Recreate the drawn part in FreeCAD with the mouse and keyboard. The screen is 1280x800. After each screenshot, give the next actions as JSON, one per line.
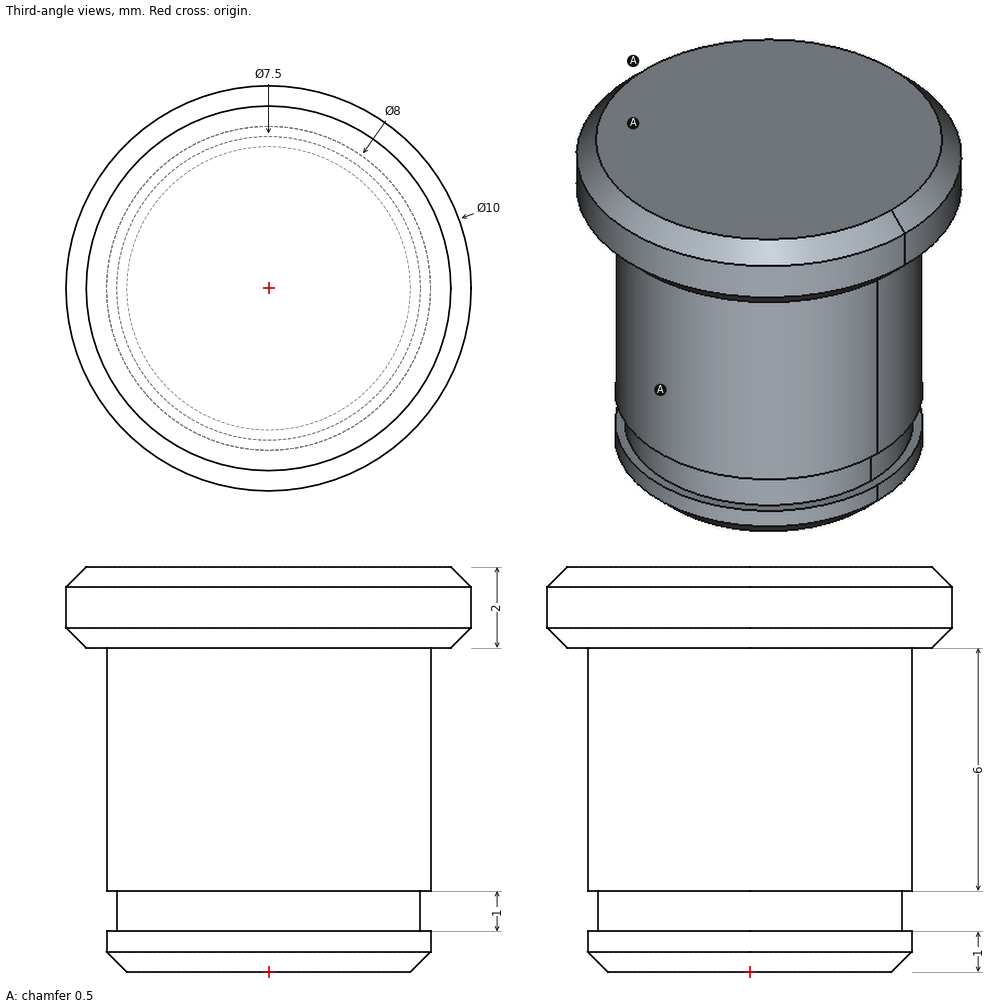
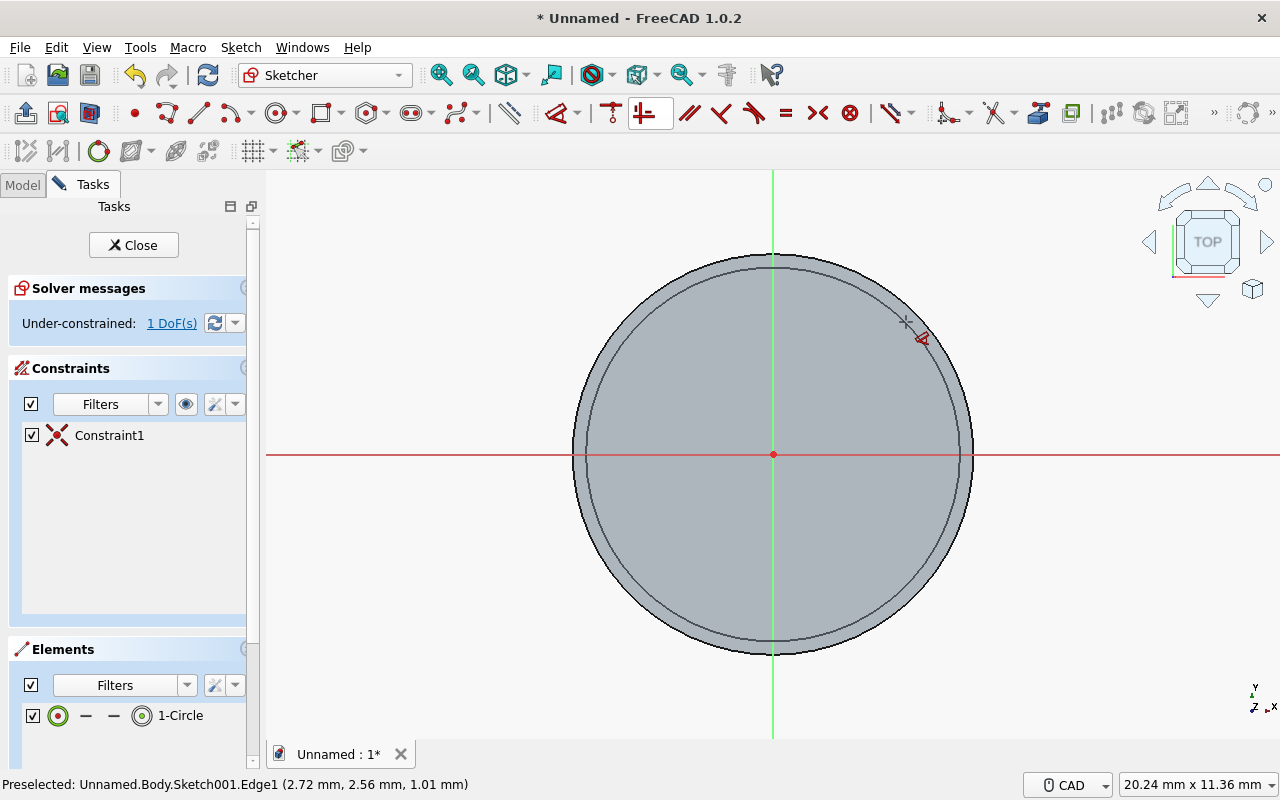
{"action": "left_click", "coordinate": [905, 322]}
{"action": "left_click", "coordinate": [928, 299]}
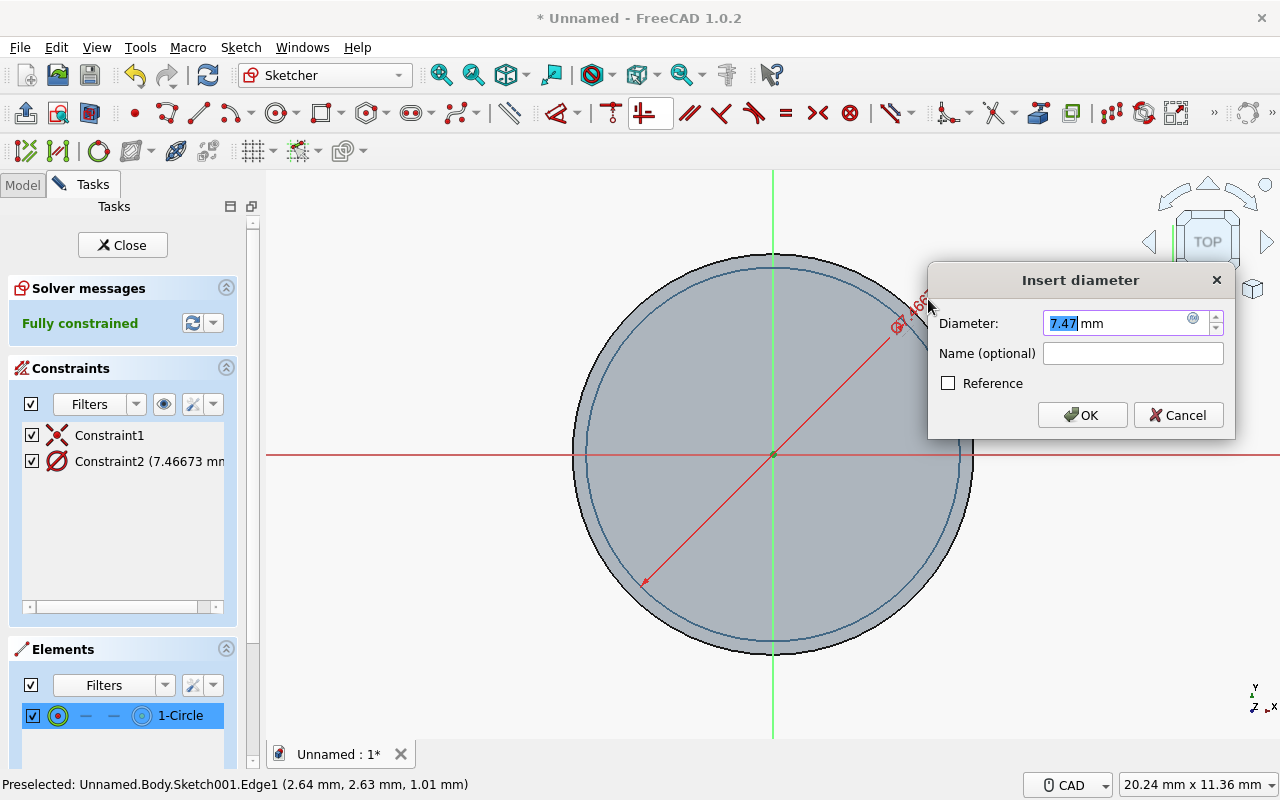
{"action": "type", "text": "7.5"}
{"action": "key", "text": "Return"}
{"action": "key", "text": "Escape"}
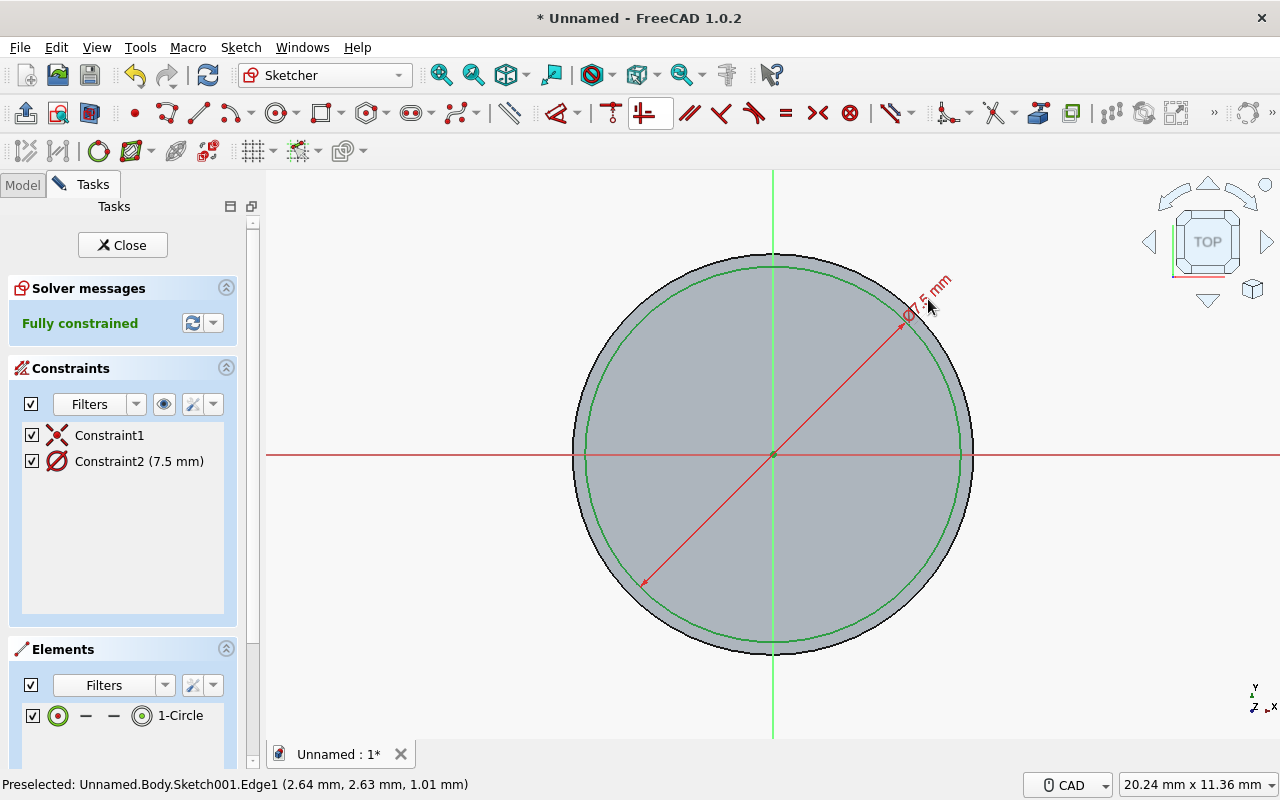
{"action": "left_click", "coordinate": [123, 245]}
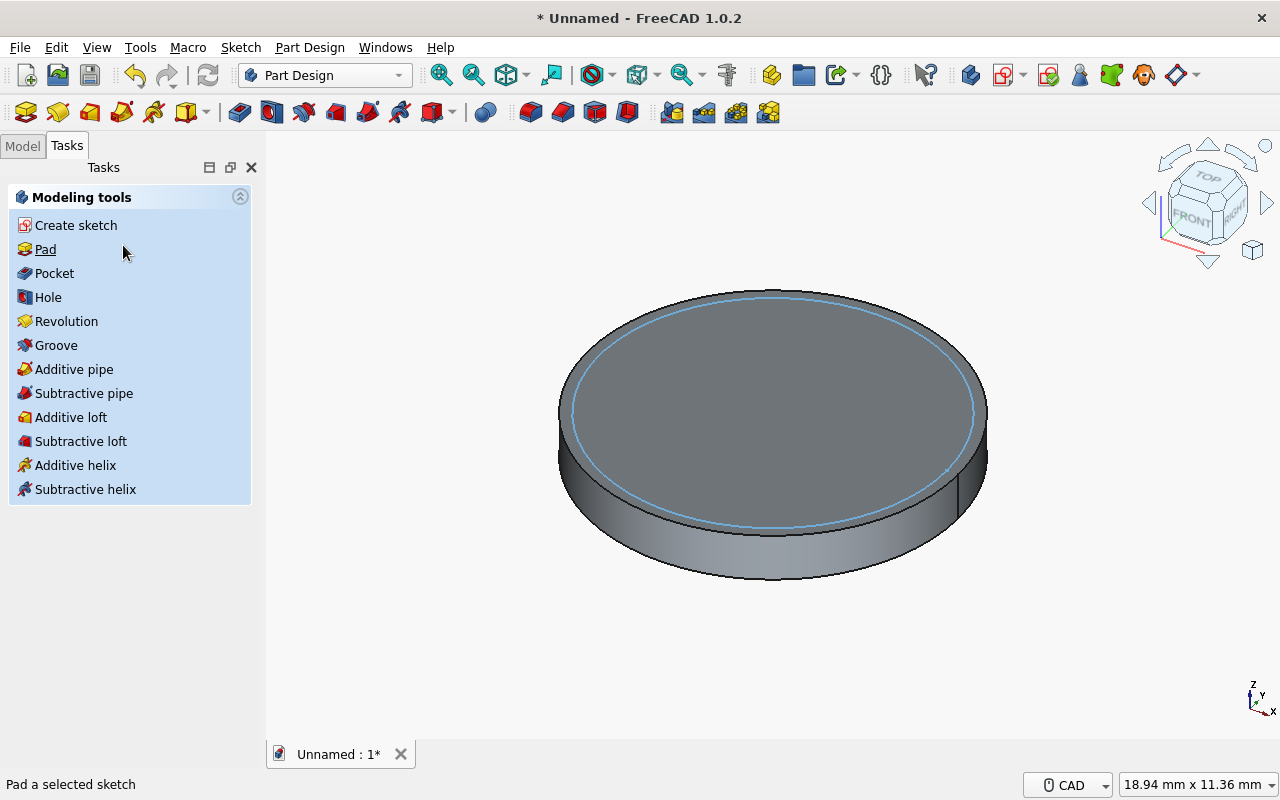
{"action": "left_click", "coordinate": [26, 112]}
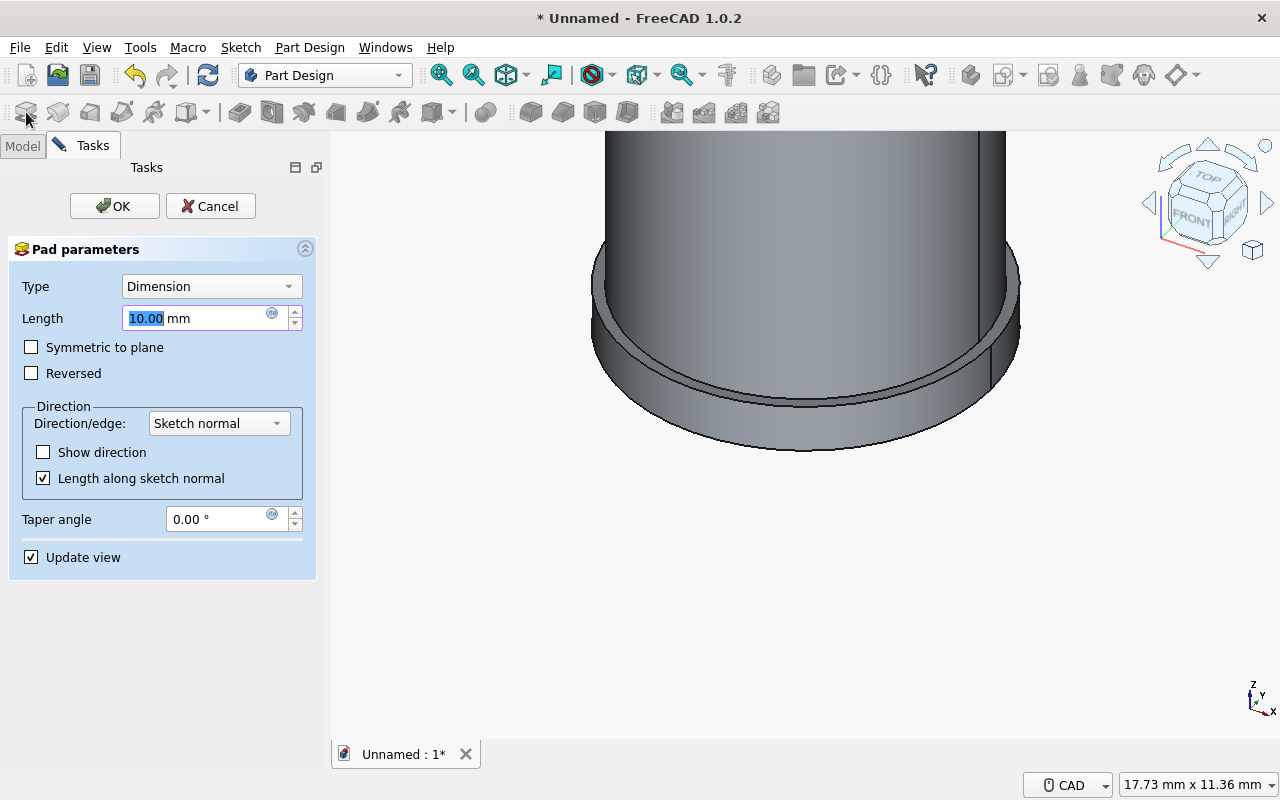
{"action": "type", "text": "1"}
{"action": "key", "text": "Tab"}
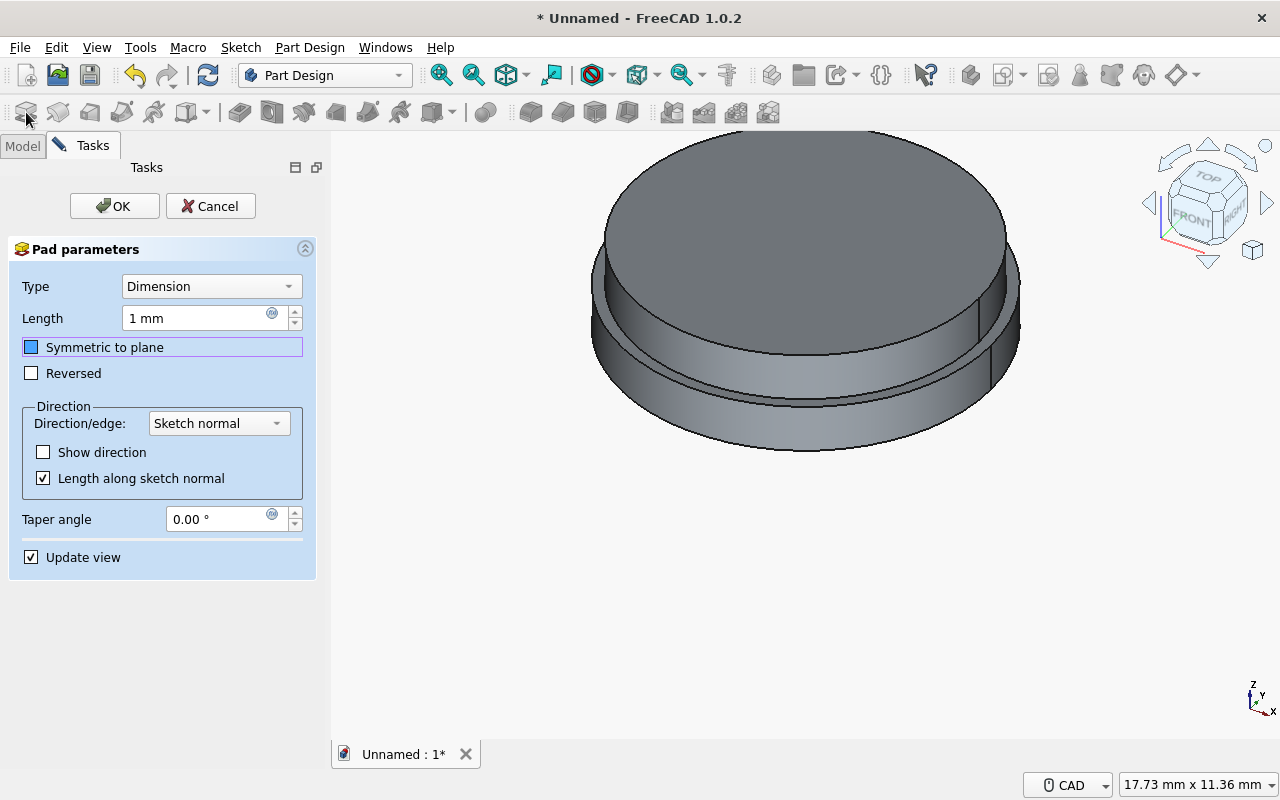
{"action": "left_click", "coordinate": [115, 206]}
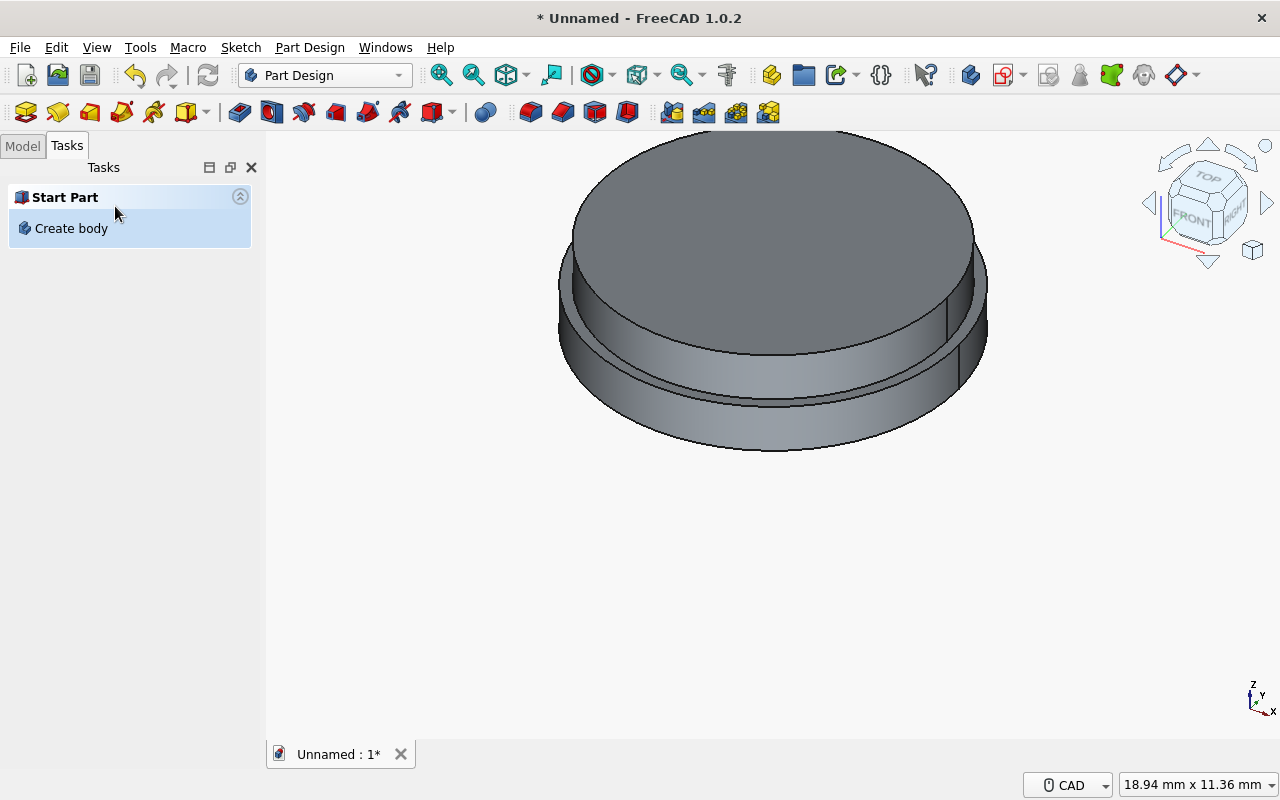
{"action": "key", "text": "v f"}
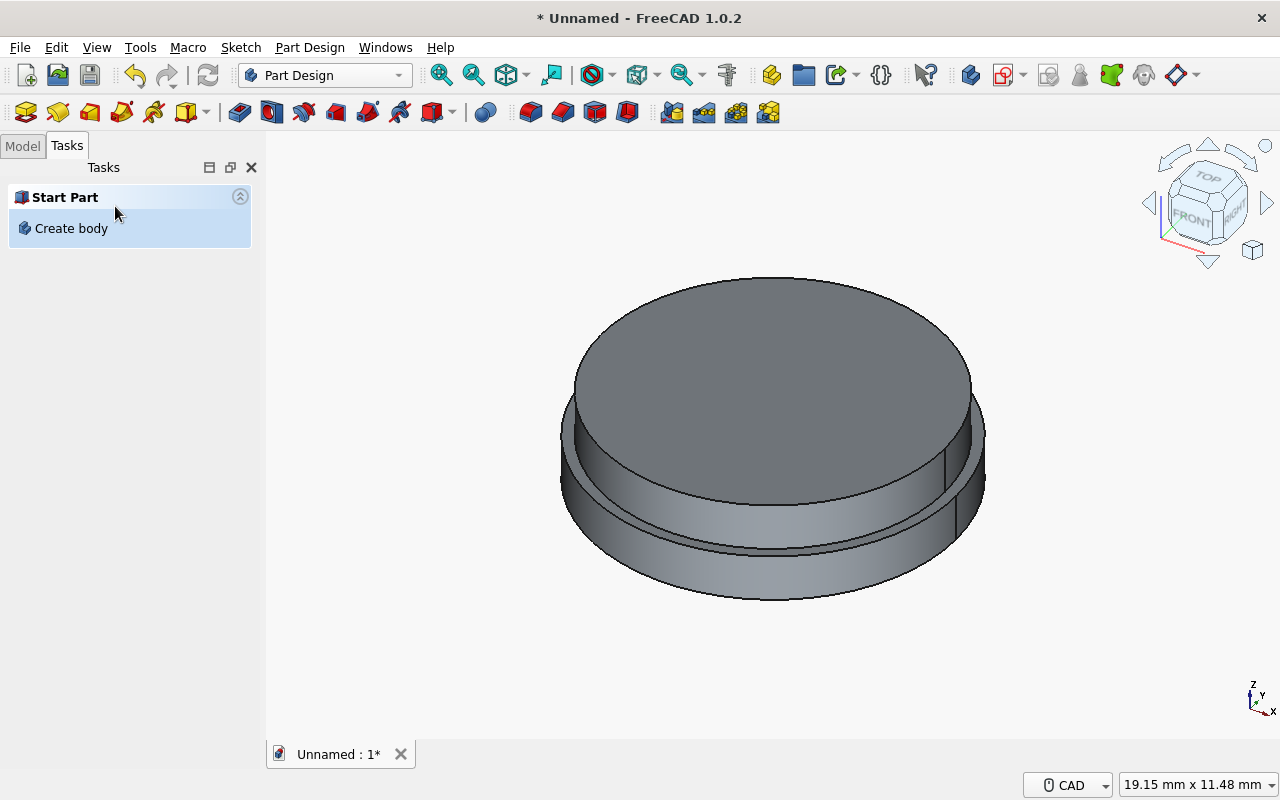
{"action": "left_click", "coordinate": [773, 391]}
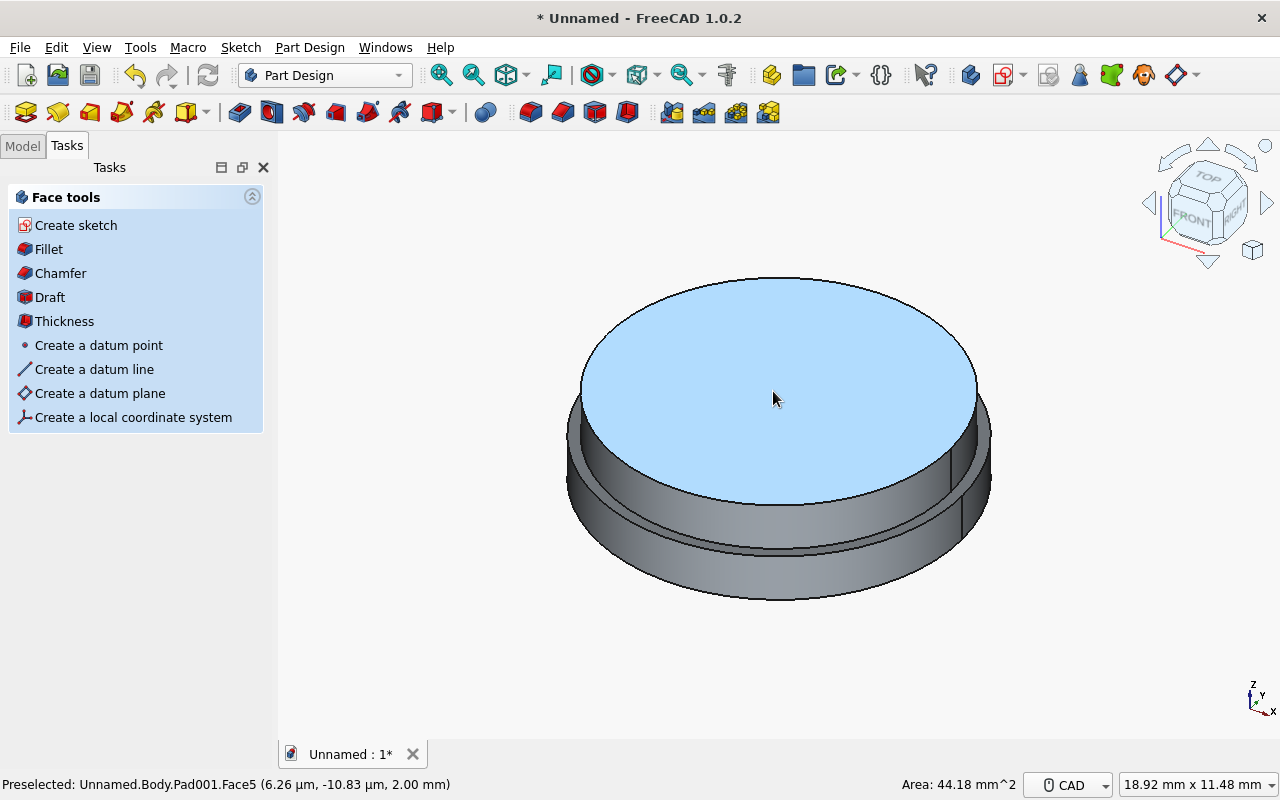
{"action": "left_click", "coordinate": [1004, 76]}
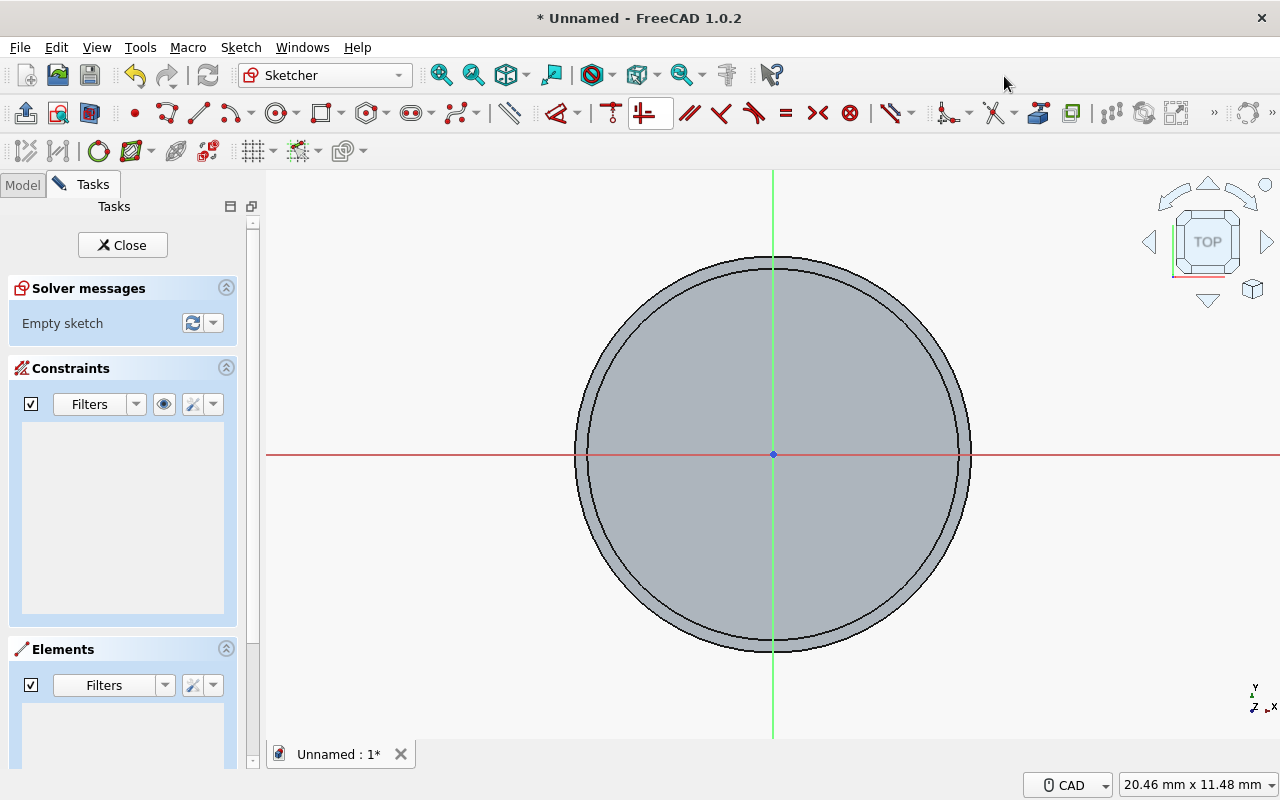
{"action": "left_click", "coordinate": [276, 114]}